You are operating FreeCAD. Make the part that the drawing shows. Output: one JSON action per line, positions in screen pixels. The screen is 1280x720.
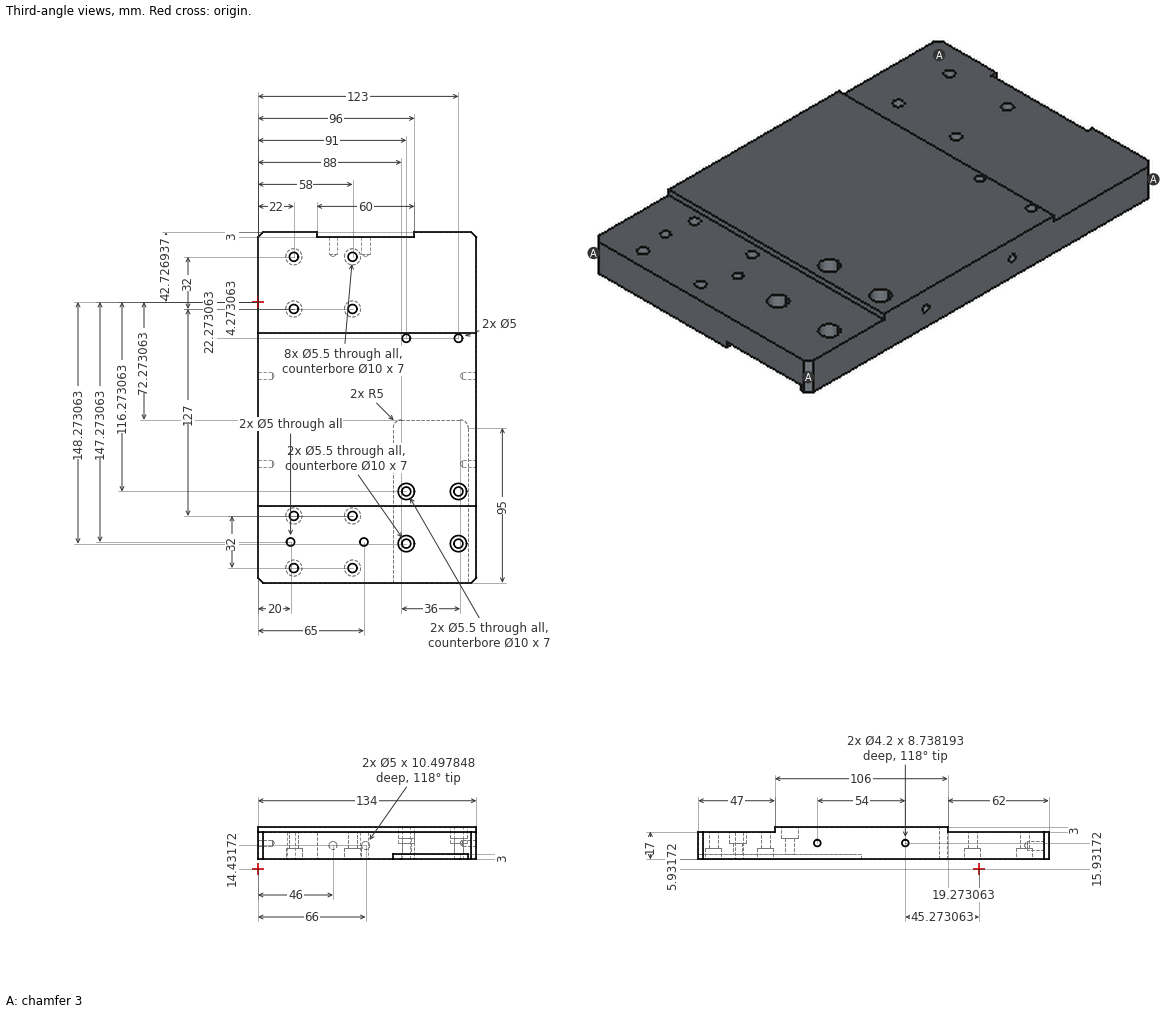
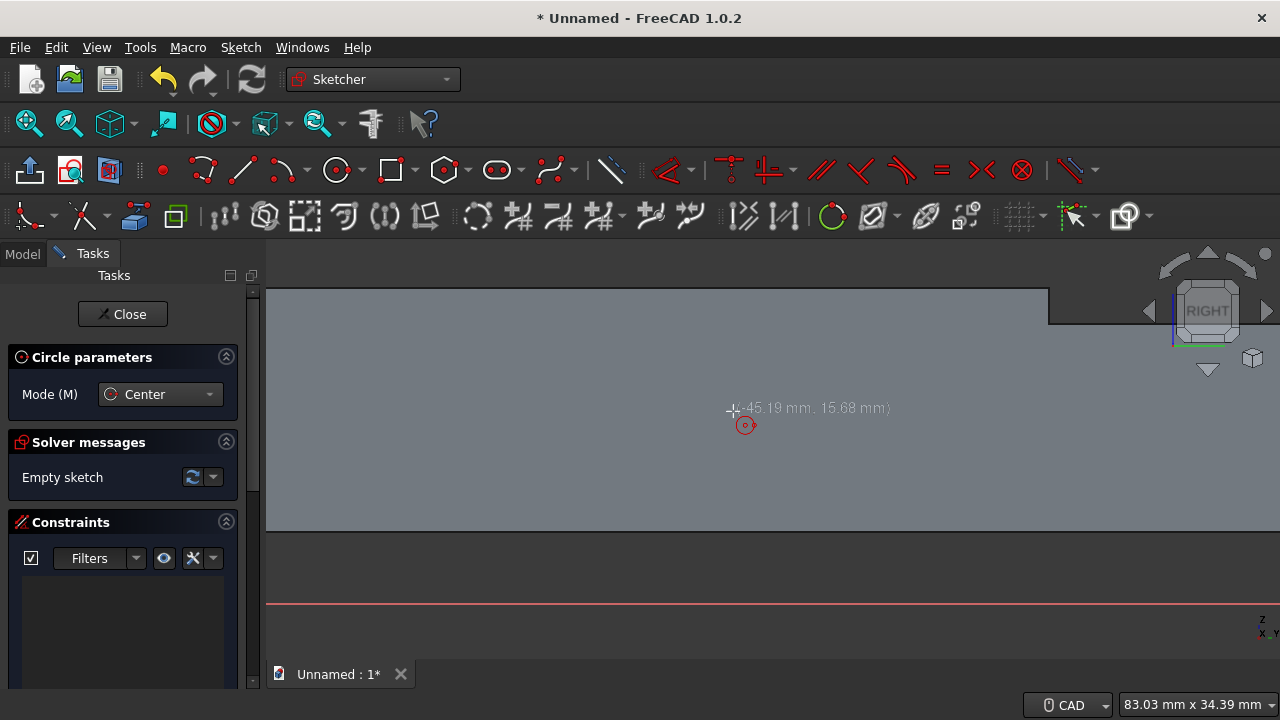
{"action": "left_click", "coordinate": [731, 410]}
{"action": "mouse_move", "coordinate": [750, 392]}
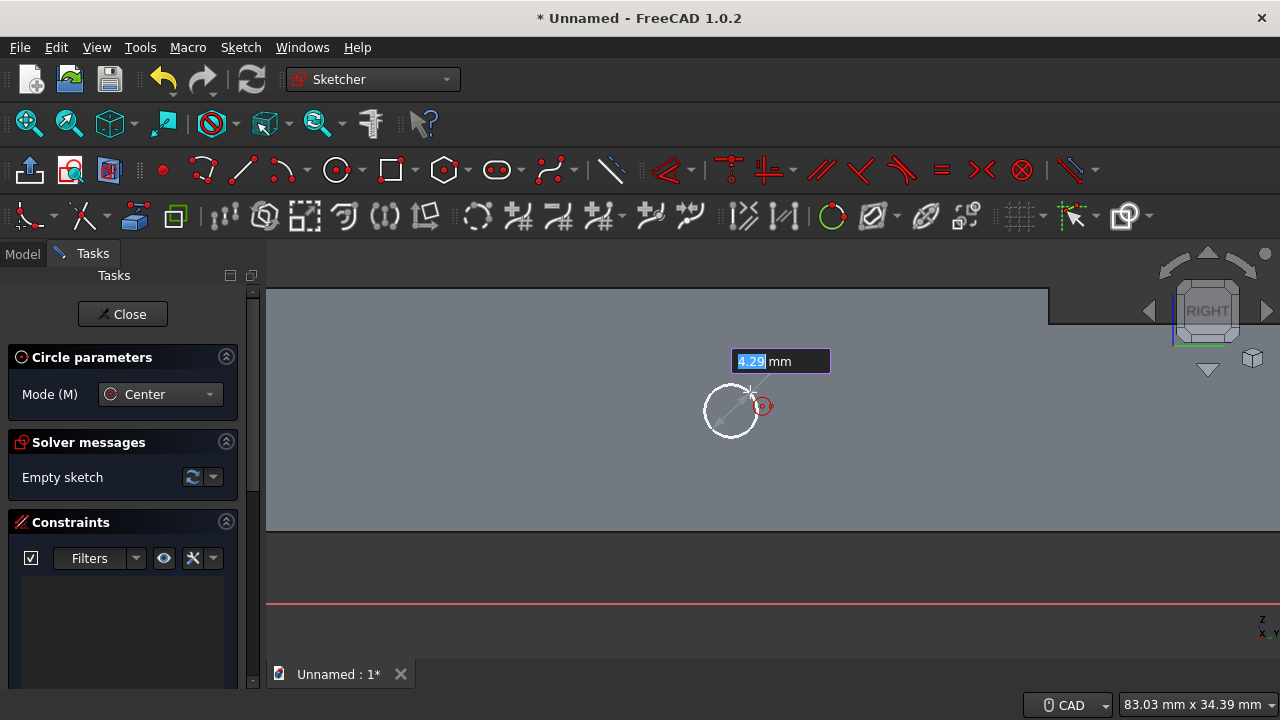
{"action": "type", "text": "4.2"}
{"action": "key", "text": "Return"}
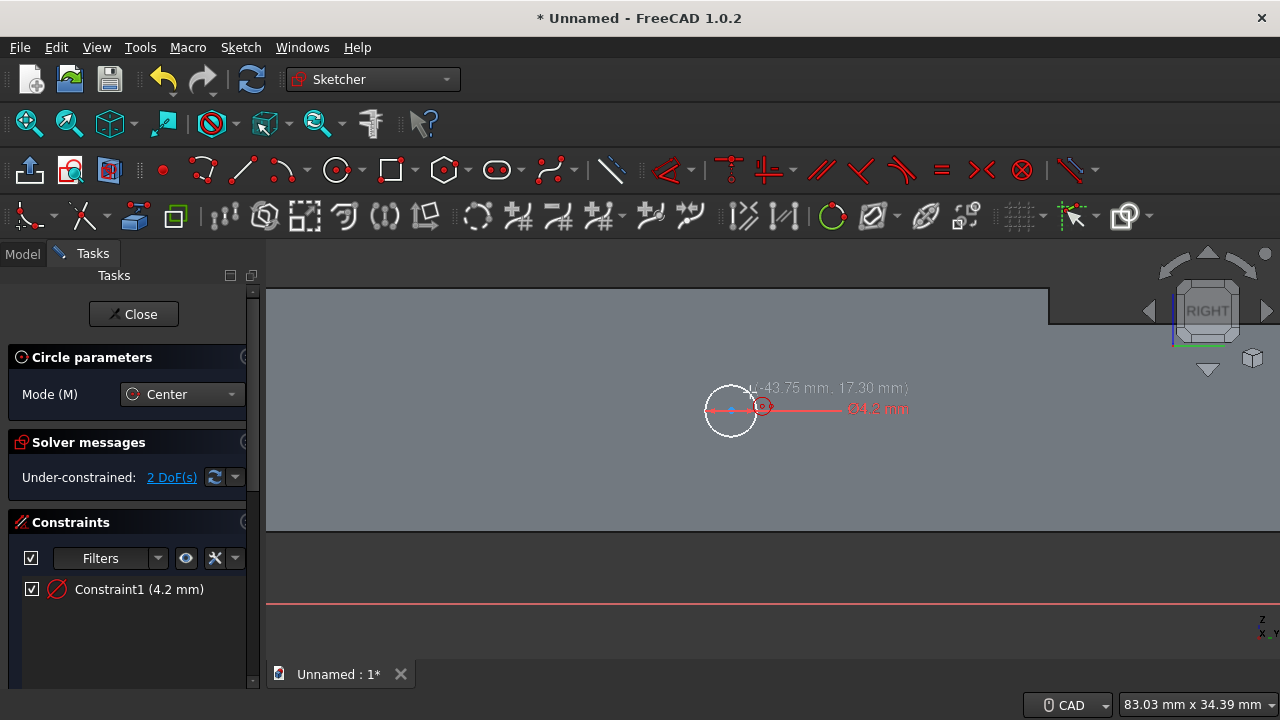
{"action": "scroll", "coordinate": [737, 412], "scroll_direction": "down", "scroll_amount": 4}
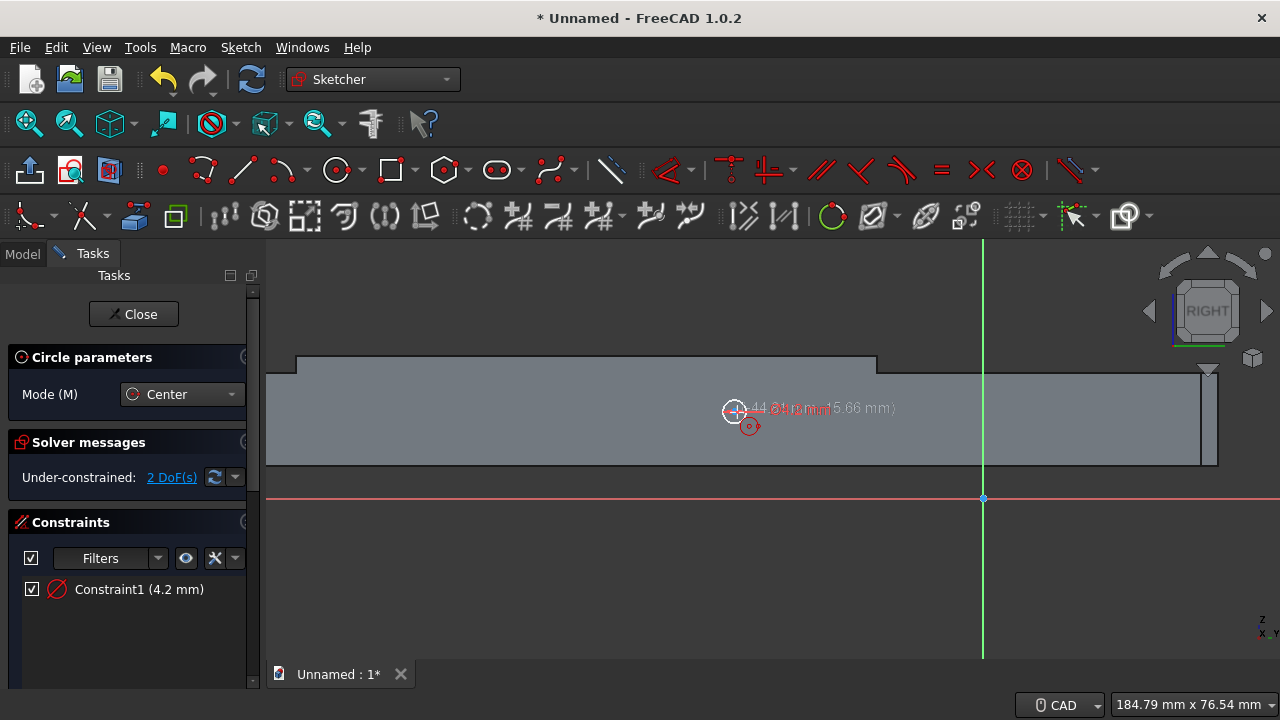
{"action": "scroll", "coordinate": [438, 411], "scroll_direction": "up", "scroll_amount": 4}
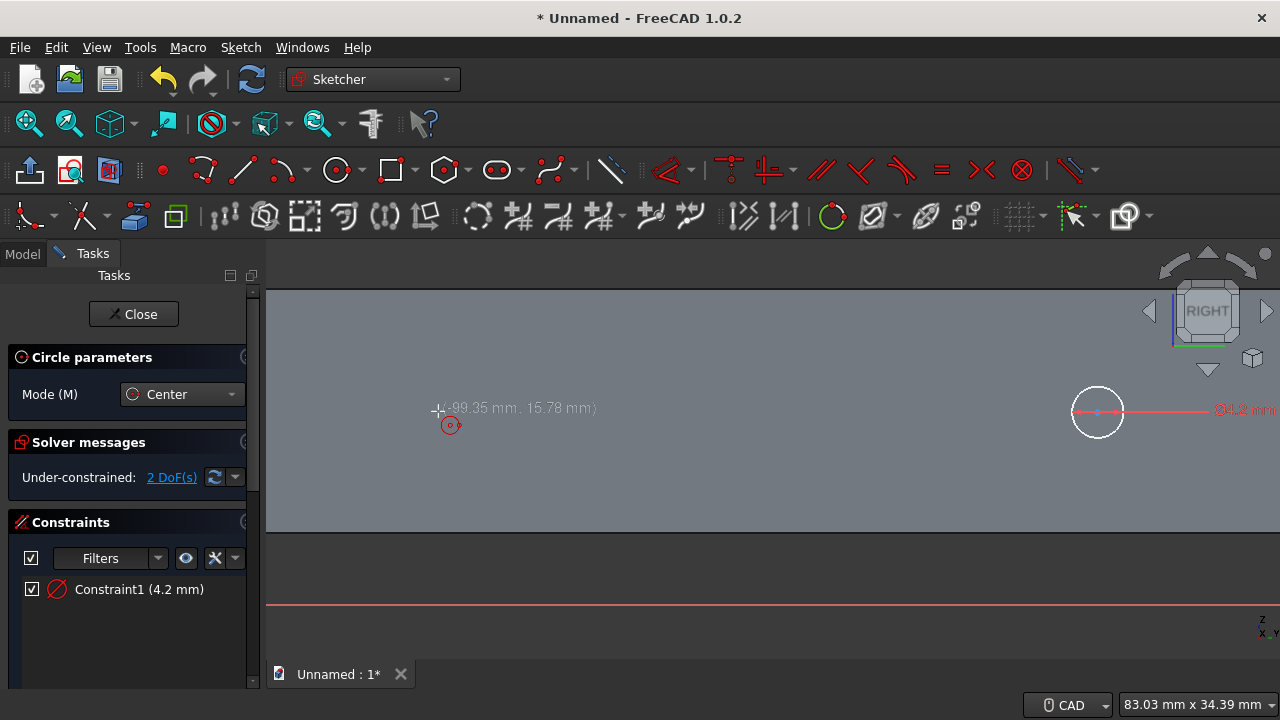
{"action": "left_click", "coordinate": [439, 411]}
{"action": "mouse_move", "coordinate": [457, 393]}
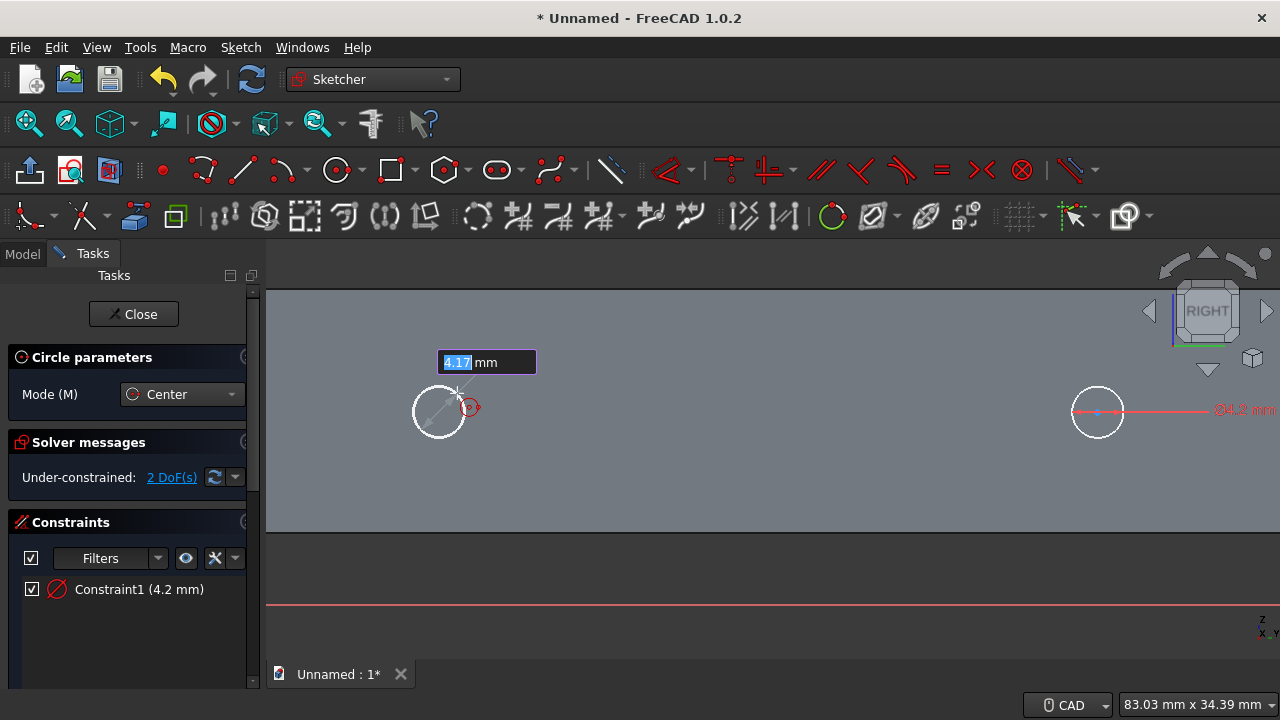
{"action": "type", "text": "4.2"}
{"action": "key", "text": "Return"}
{"action": "key", "text": "Escape"}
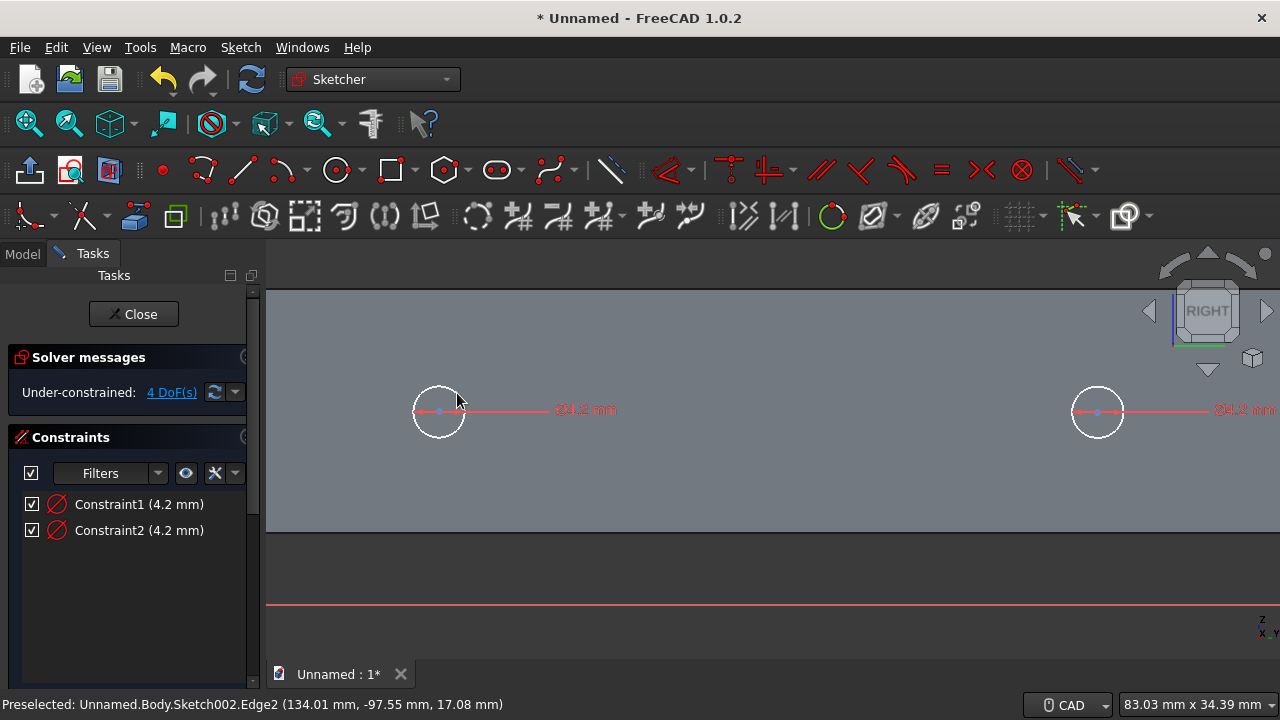
{"action": "left_click", "coordinate": [1098, 412]}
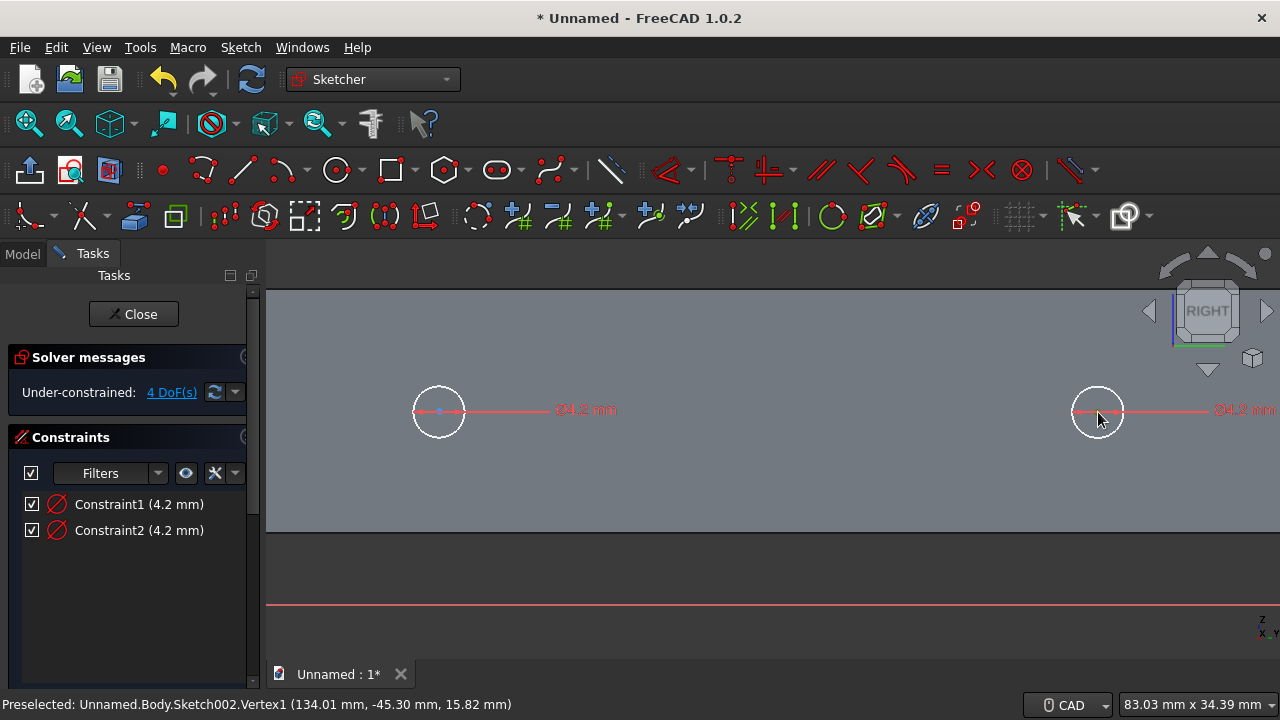
{"action": "left_click", "coordinate": [439, 412]}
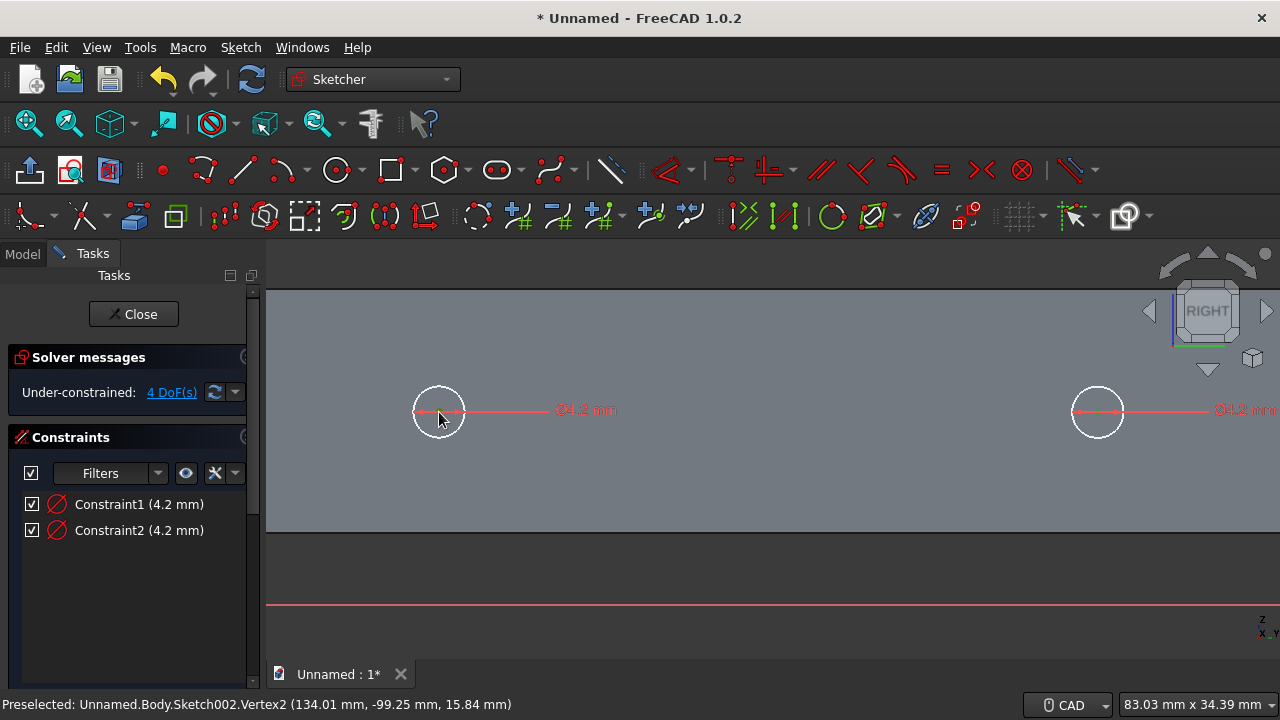
{"action": "left_click", "coordinate": [796, 170]}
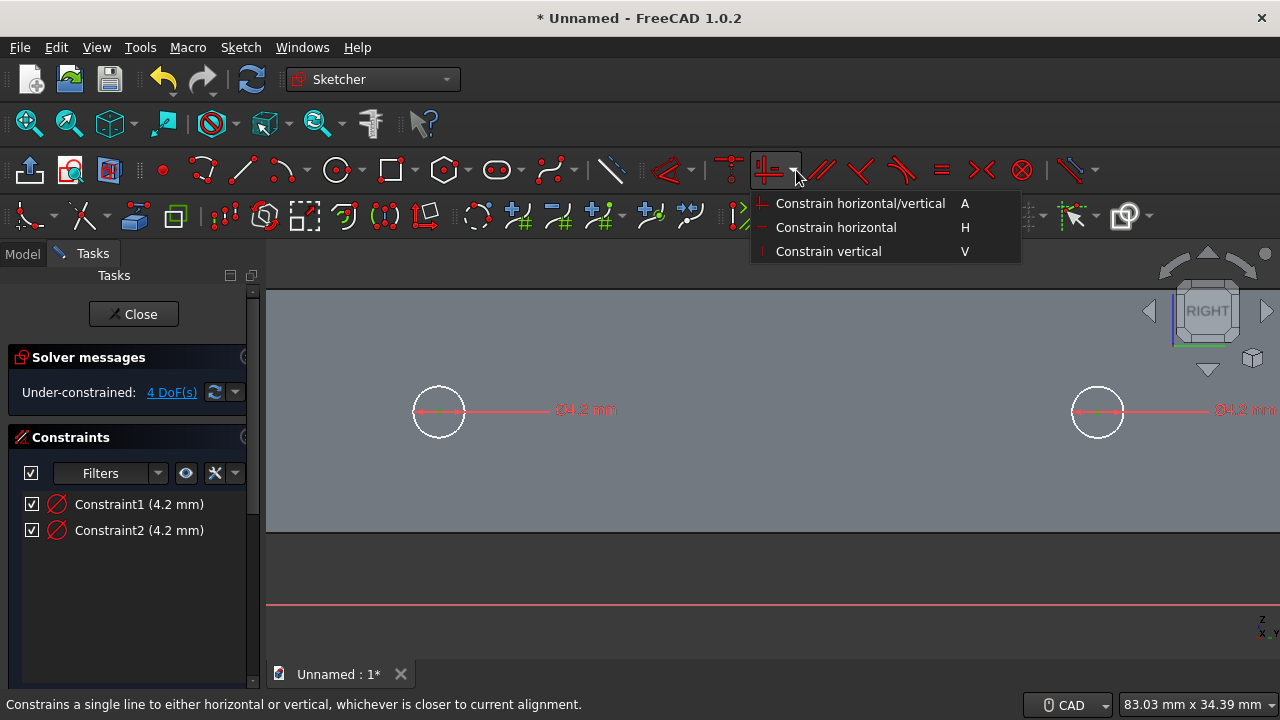
{"action": "left_click", "coordinate": [886, 227]}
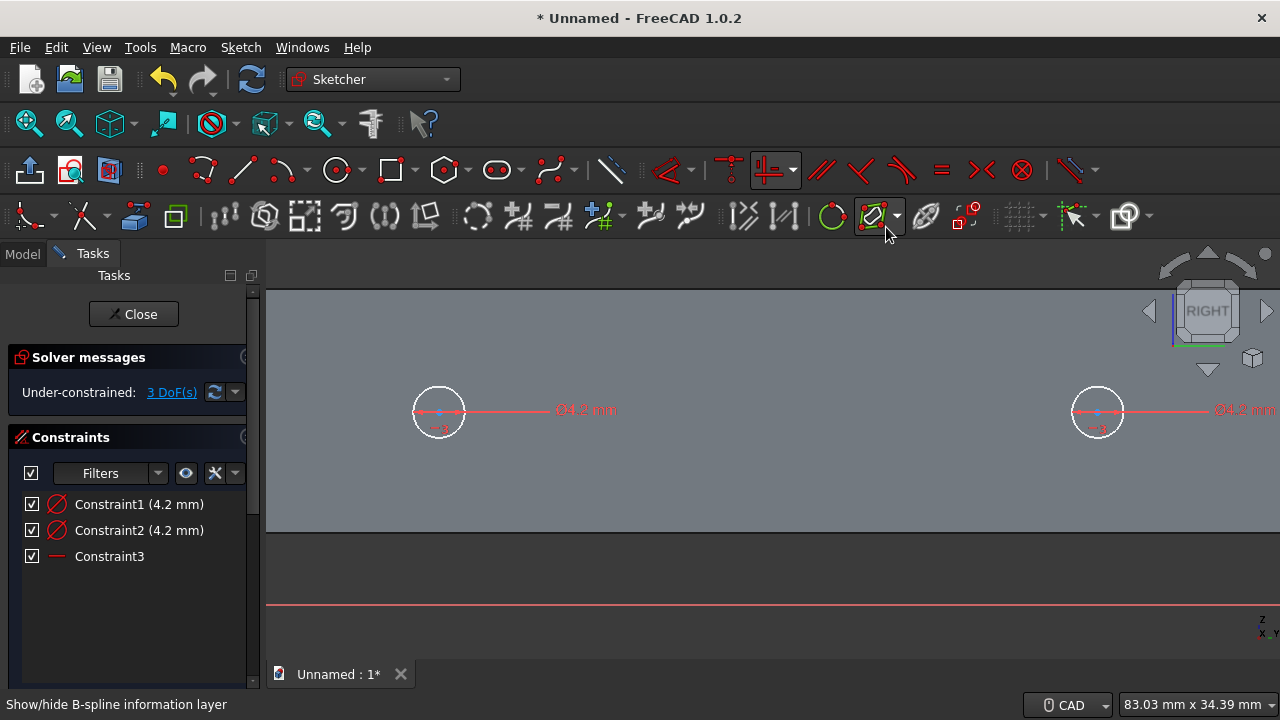
{"action": "left_click", "coordinate": [666, 170]}